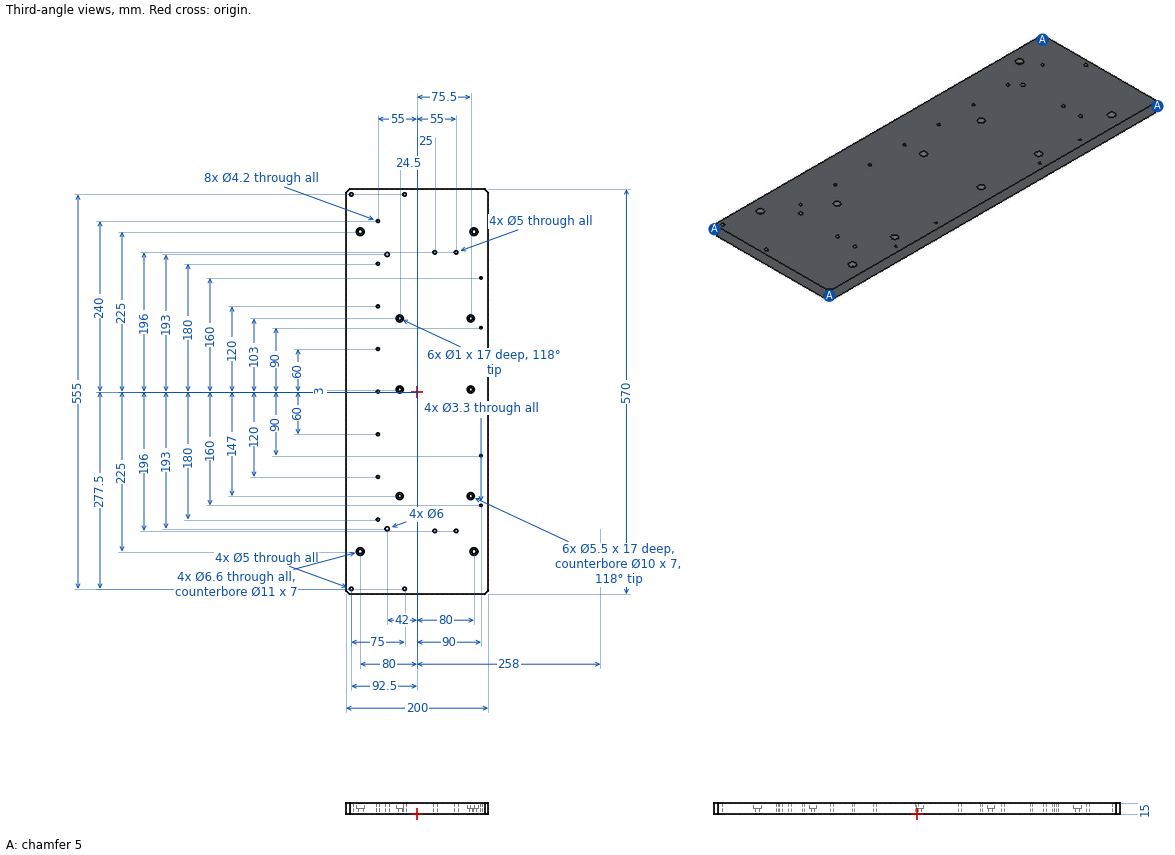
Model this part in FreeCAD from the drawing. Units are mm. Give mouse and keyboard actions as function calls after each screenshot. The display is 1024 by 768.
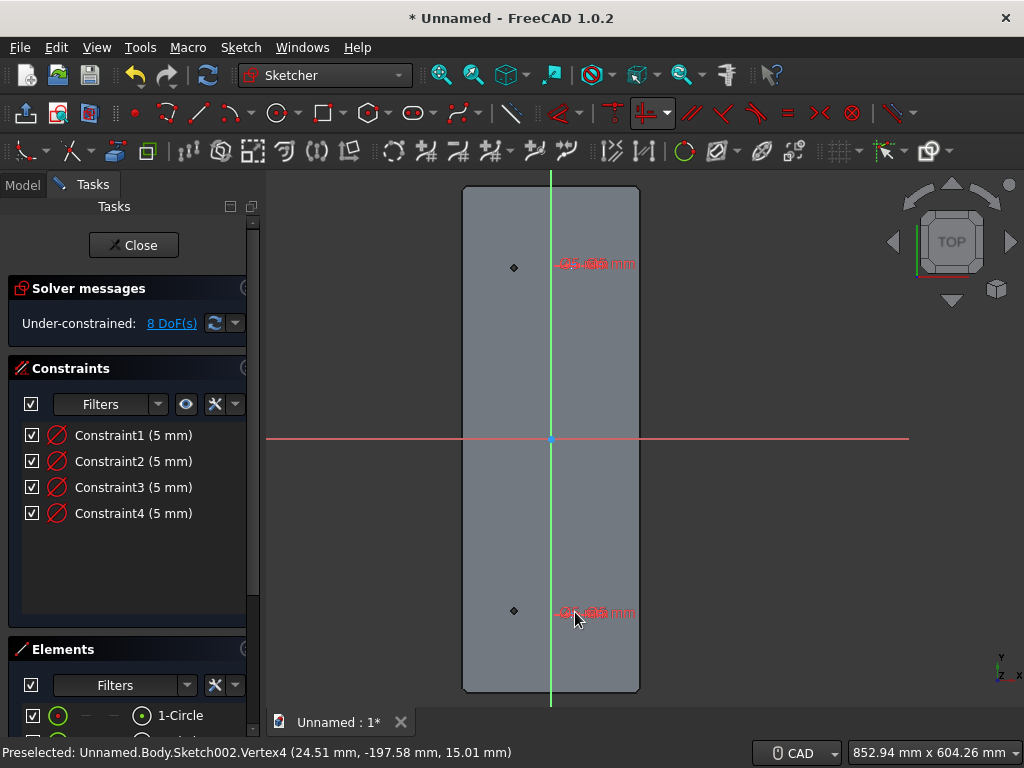
click(600, 266)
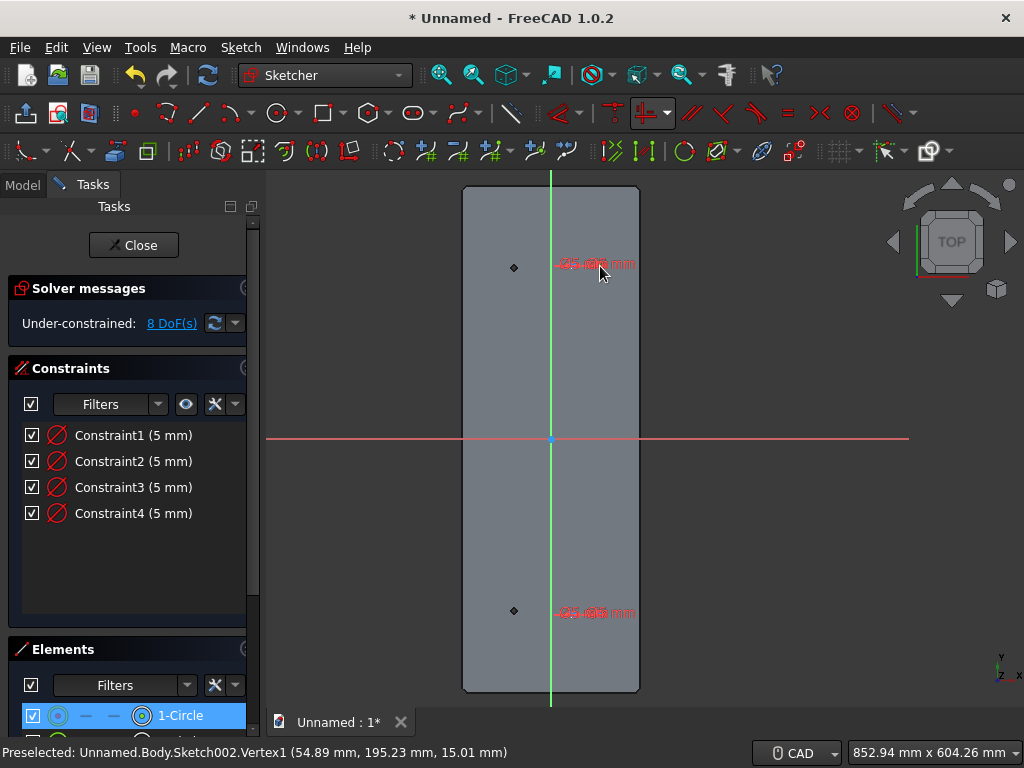
click(573, 266)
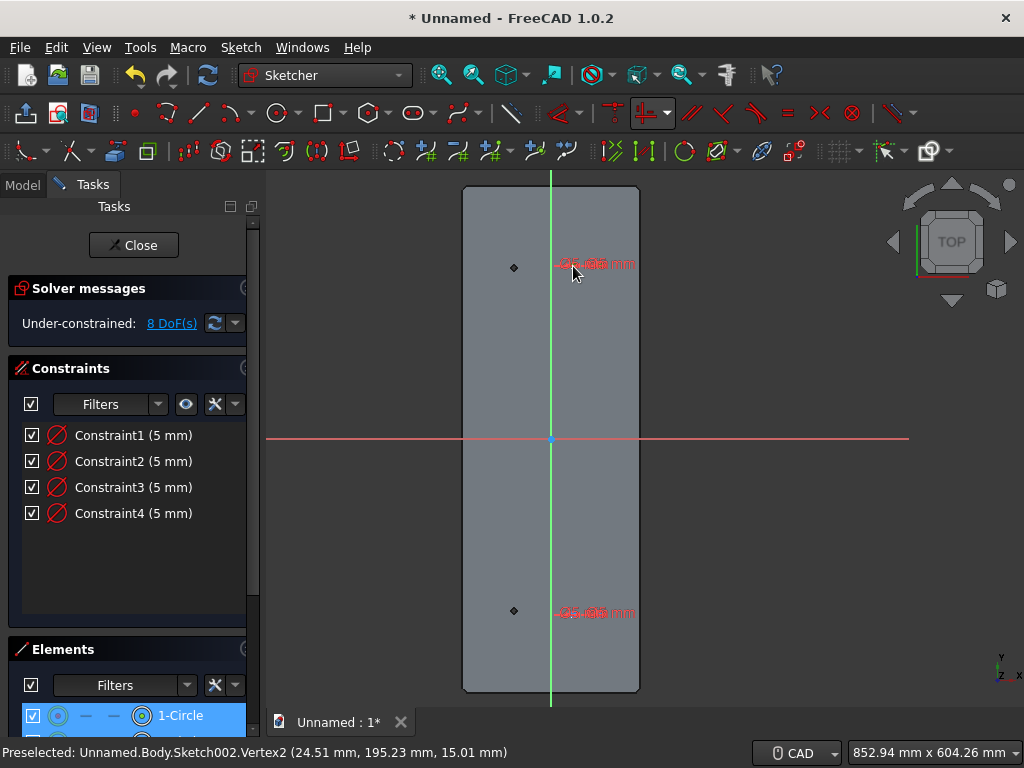
click(670, 114)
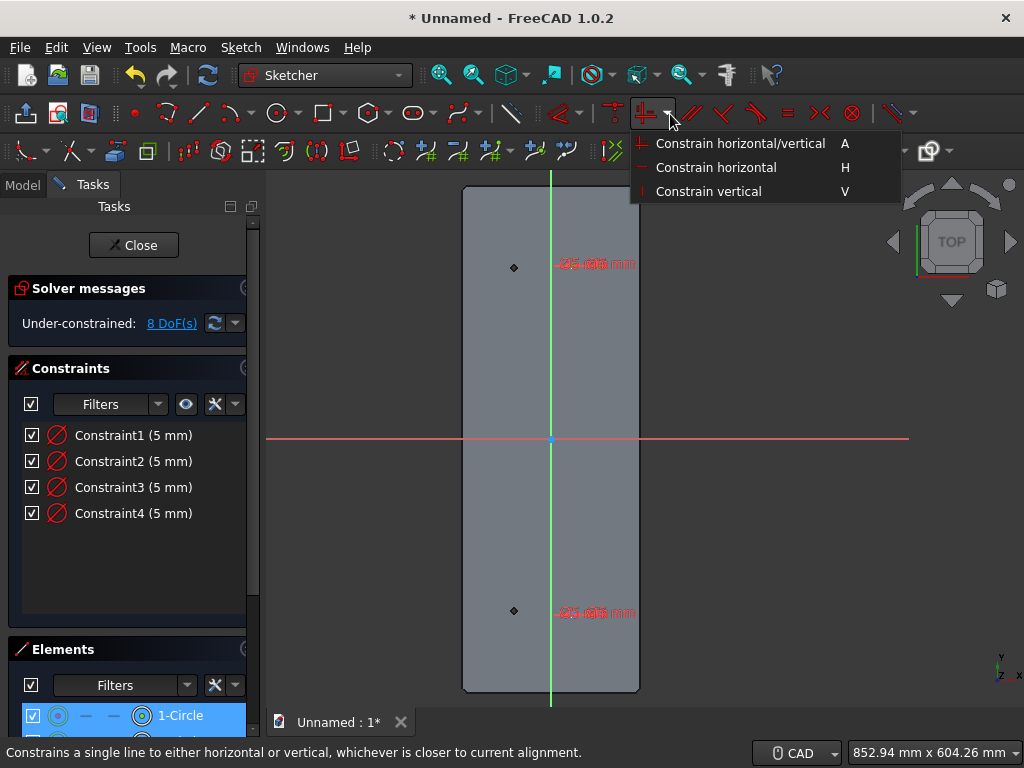
click(766, 167)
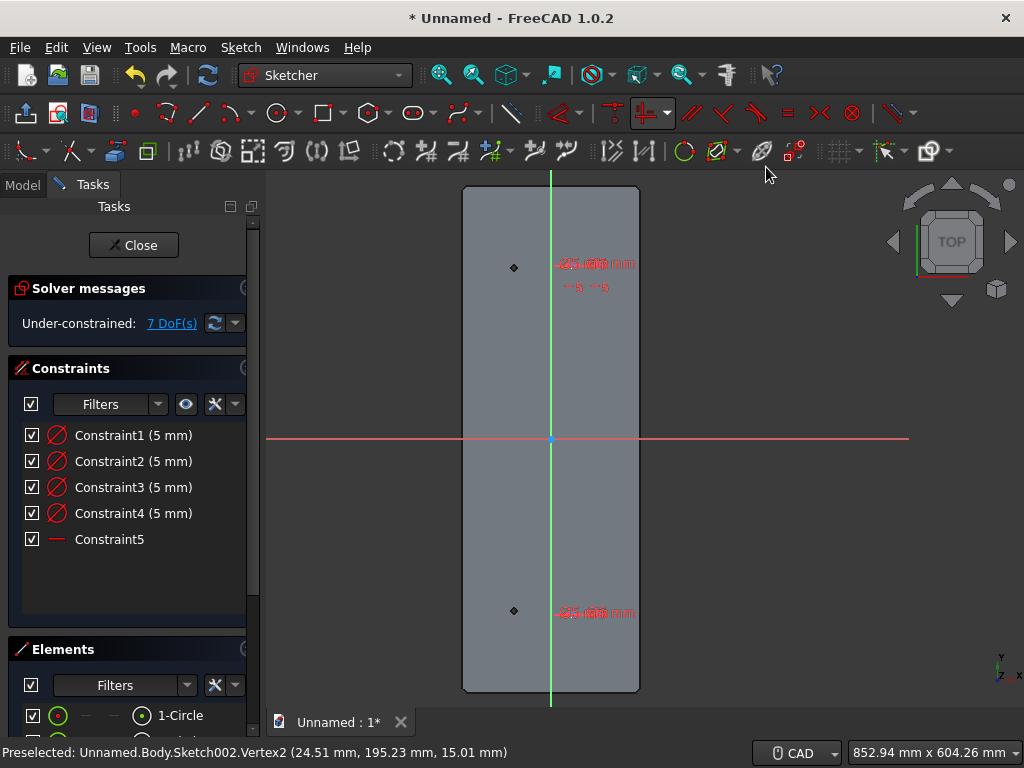
click(600, 266)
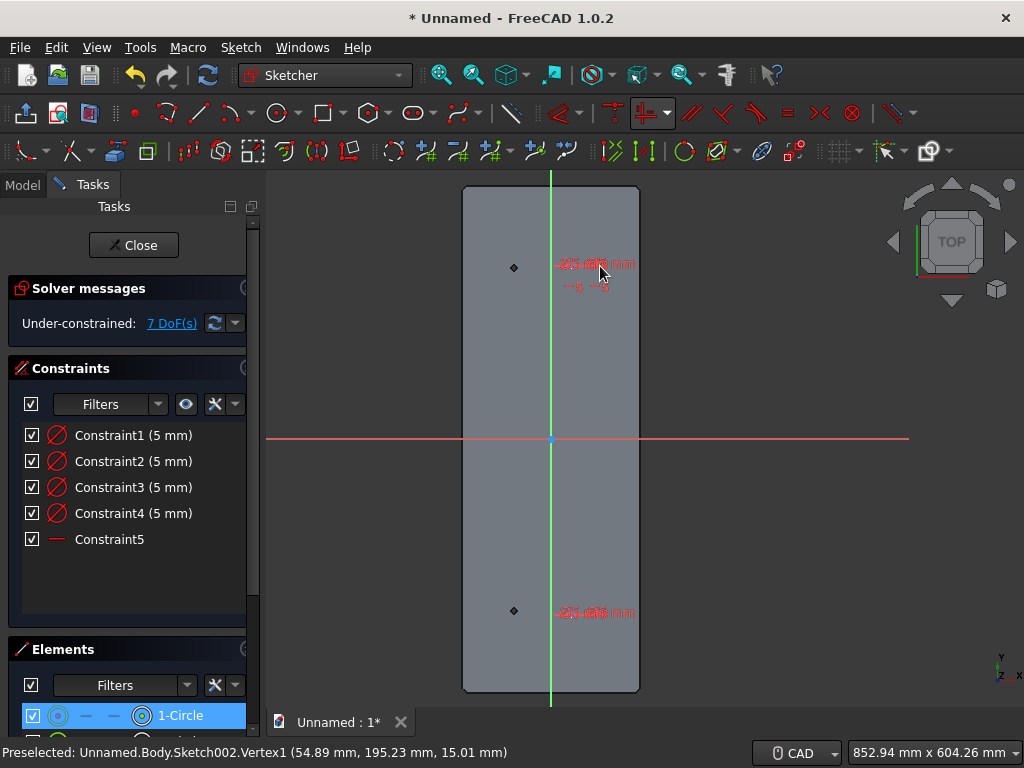
click(600, 615)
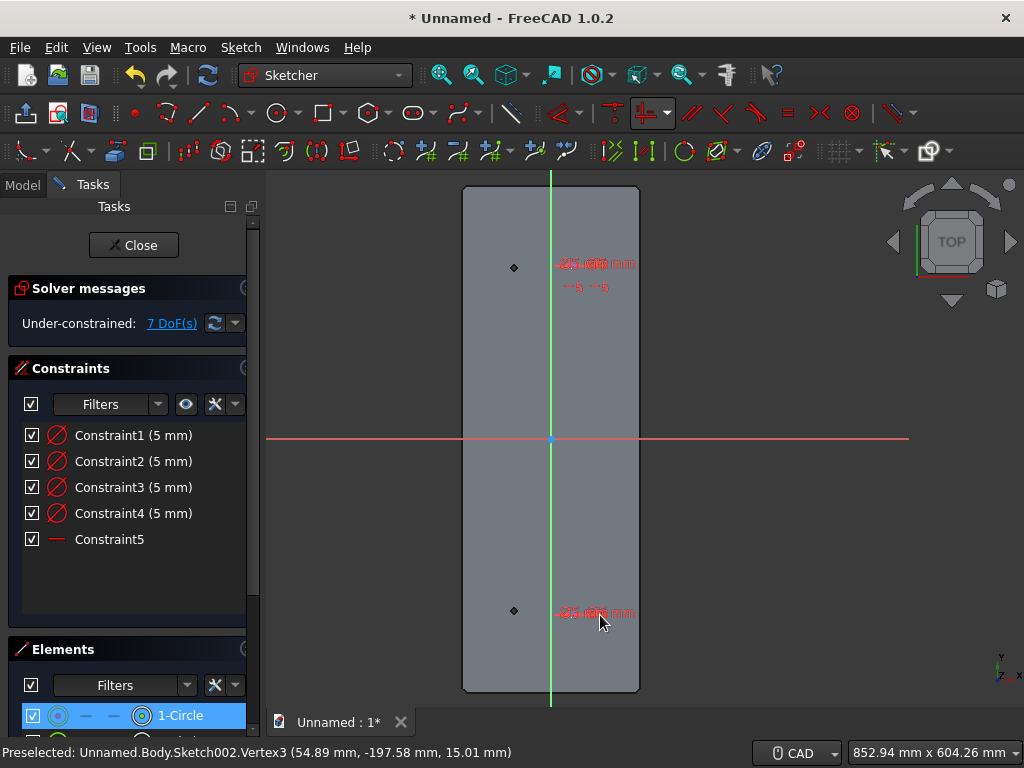
click(670, 114)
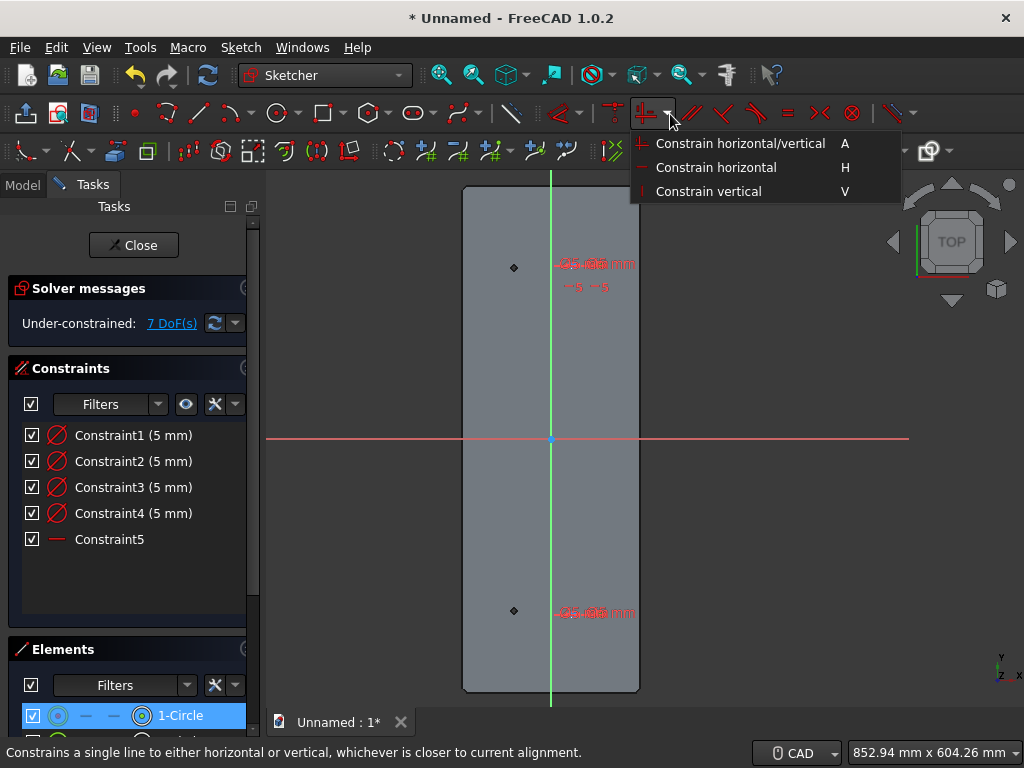
click(766, 191)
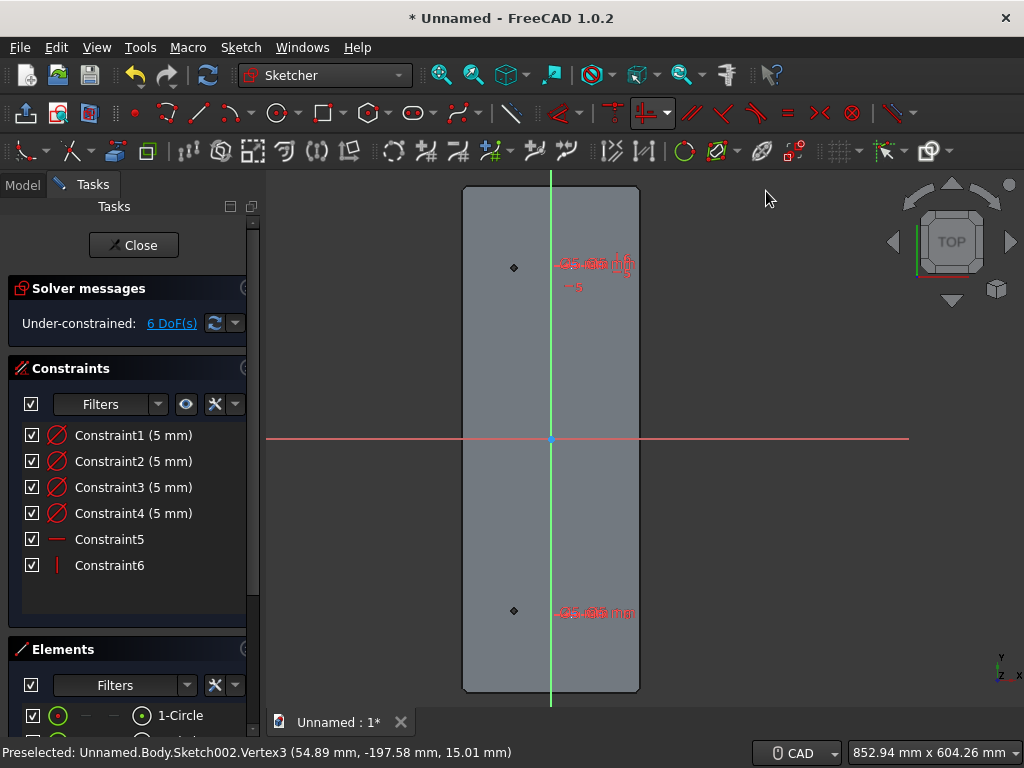
click(573, 266)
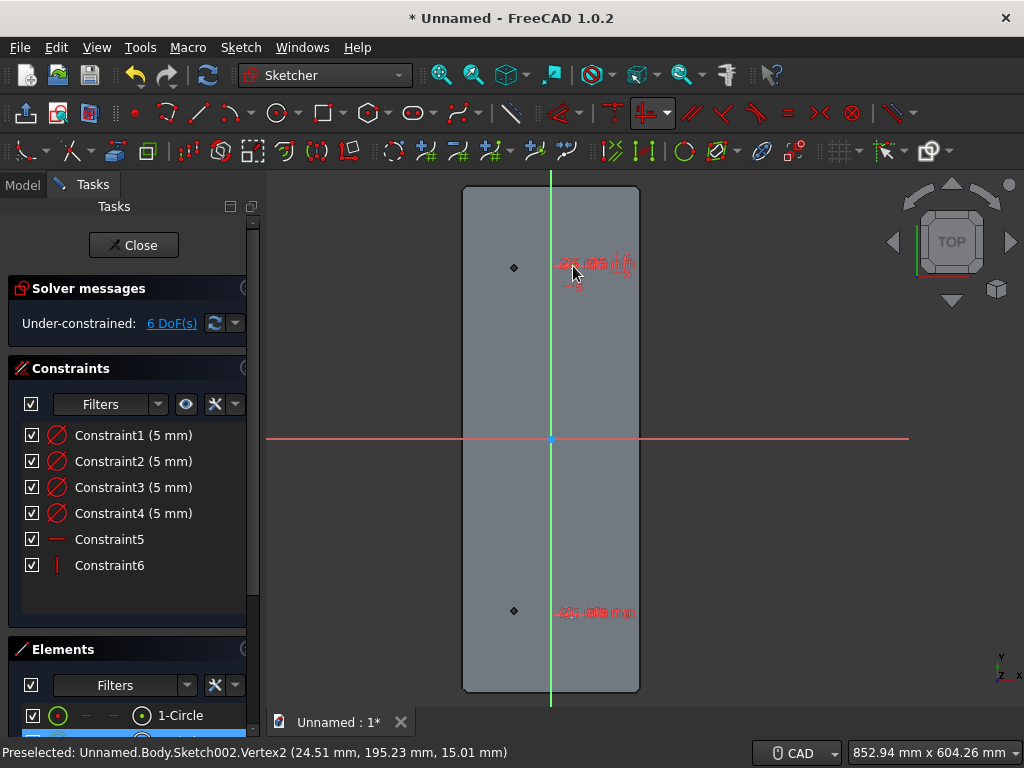
click(573, 615)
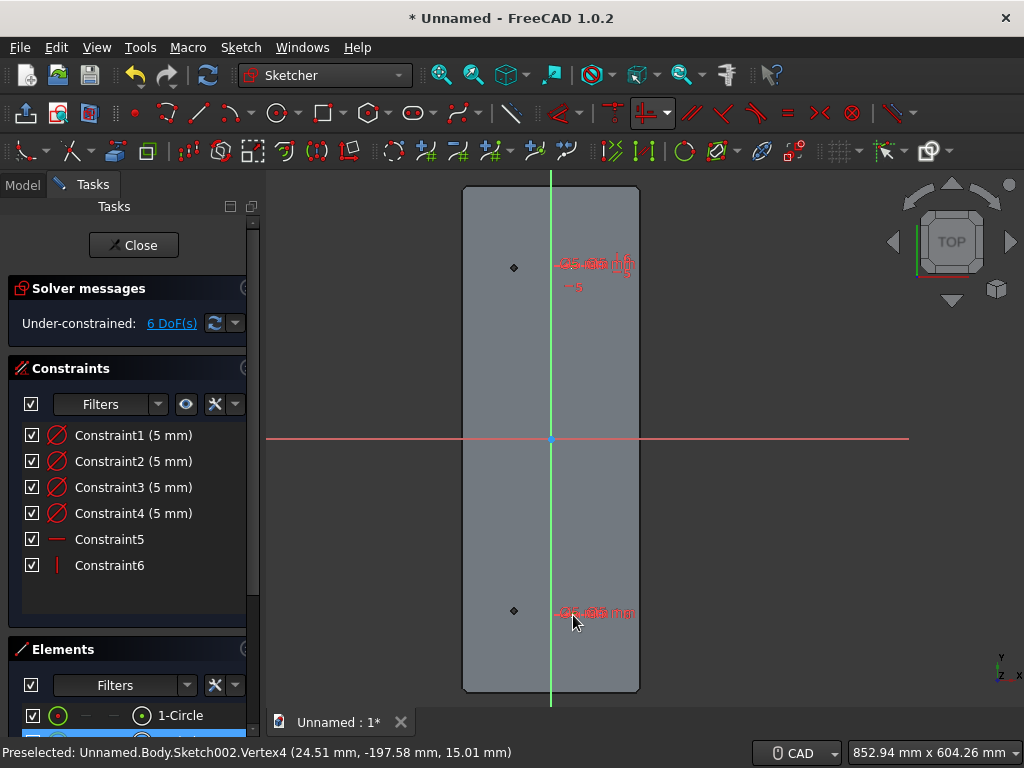
key(v)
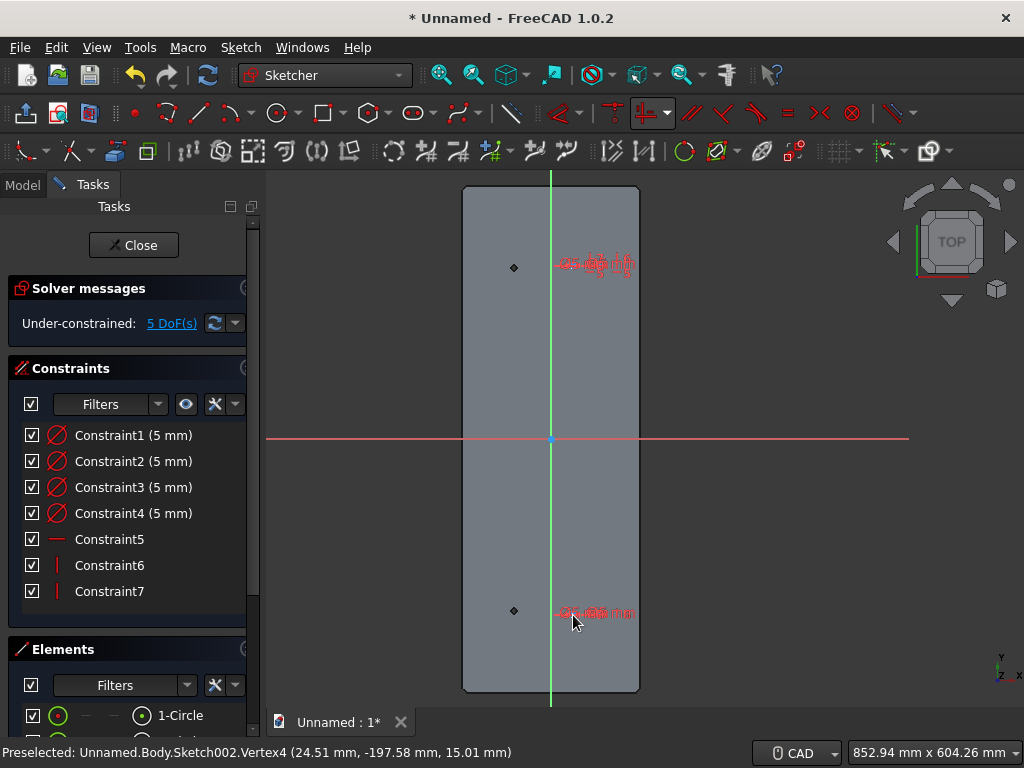
scroll(600, 615, up, 4)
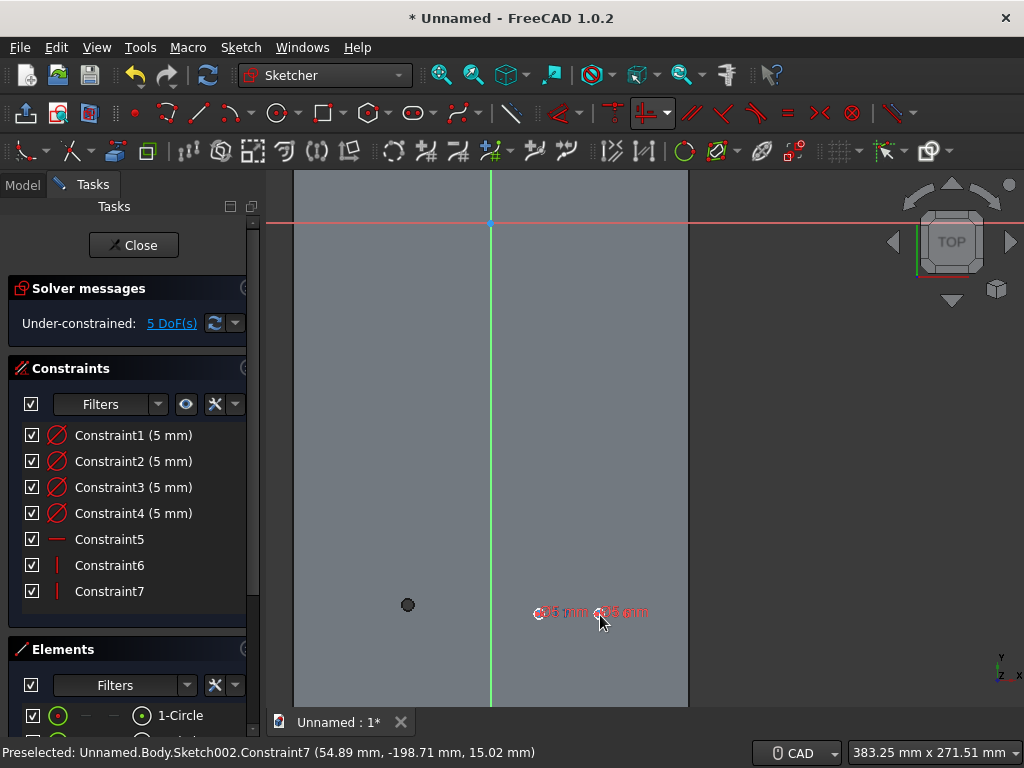
click(599, 614)